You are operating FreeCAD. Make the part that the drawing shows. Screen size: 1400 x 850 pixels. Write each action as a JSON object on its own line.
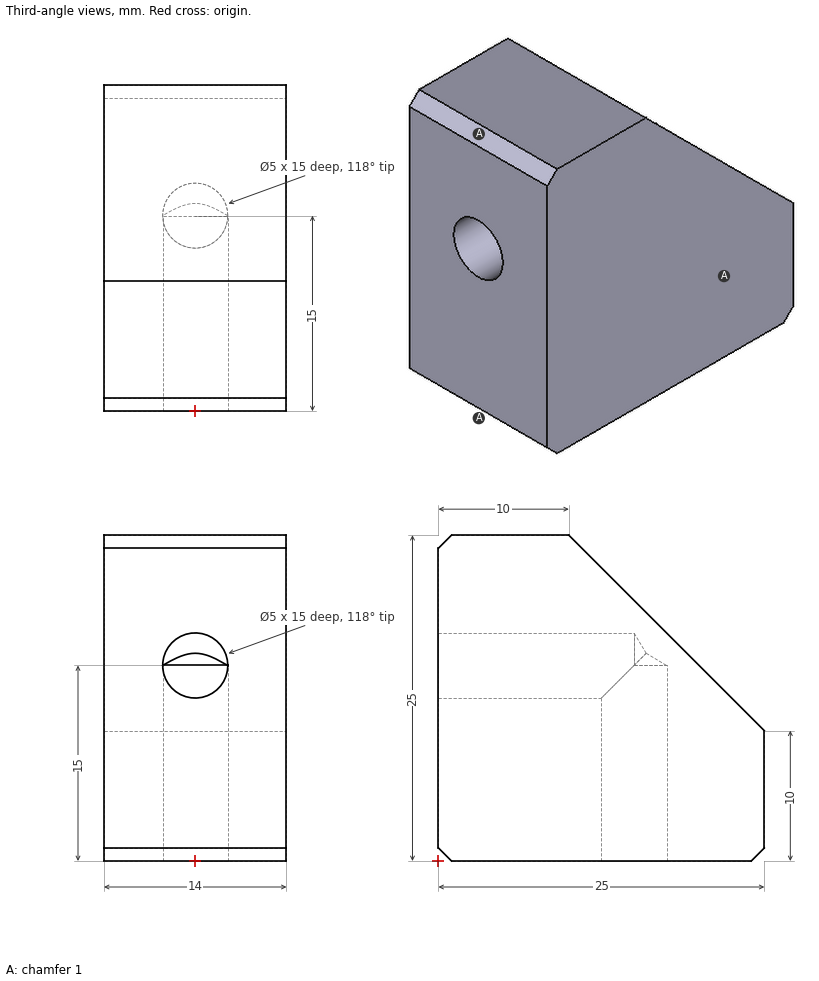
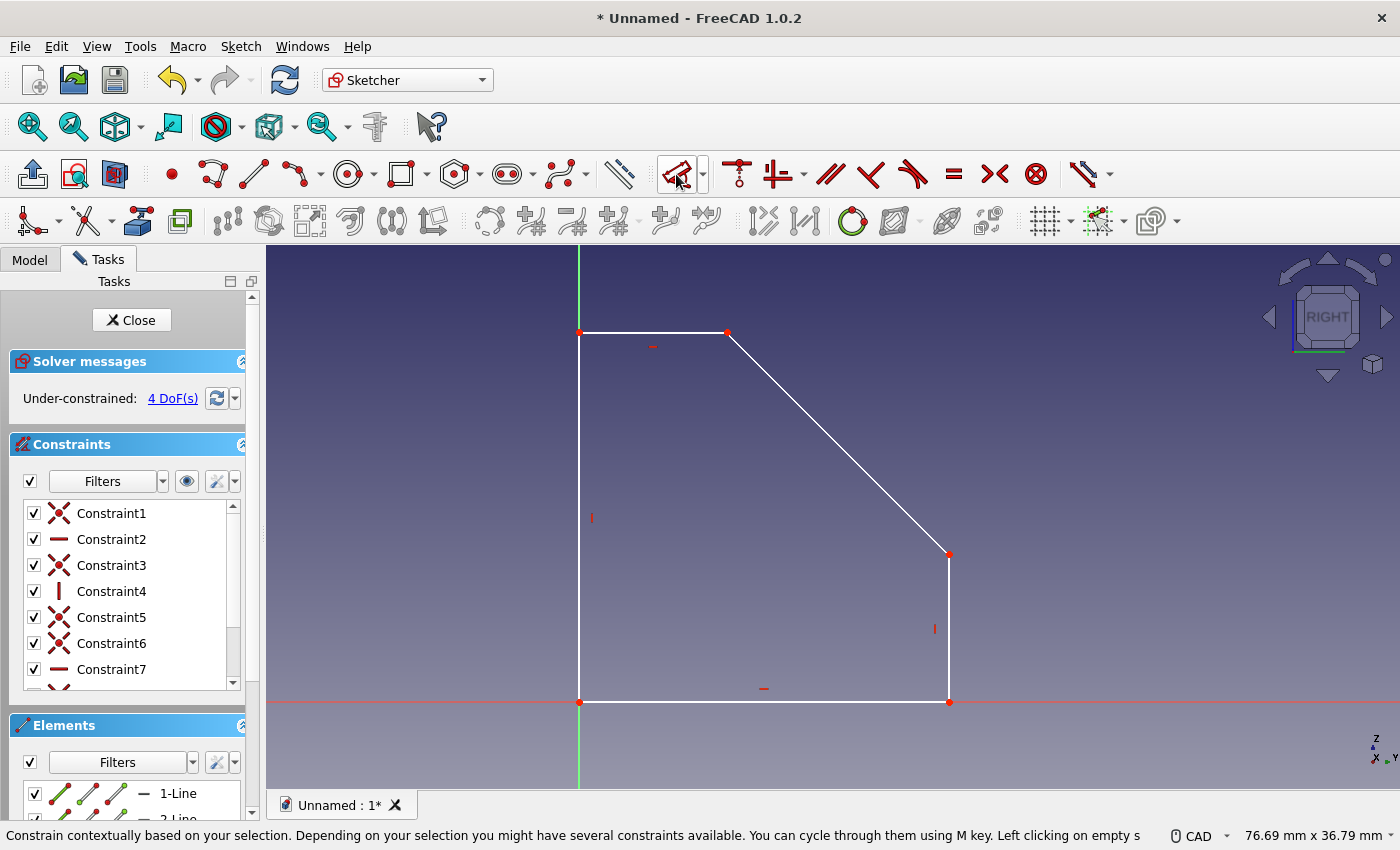
{"action": "left_click", "coordinate": [690, 702]}
{"action": "left_click", "coordinate": [764, 736]}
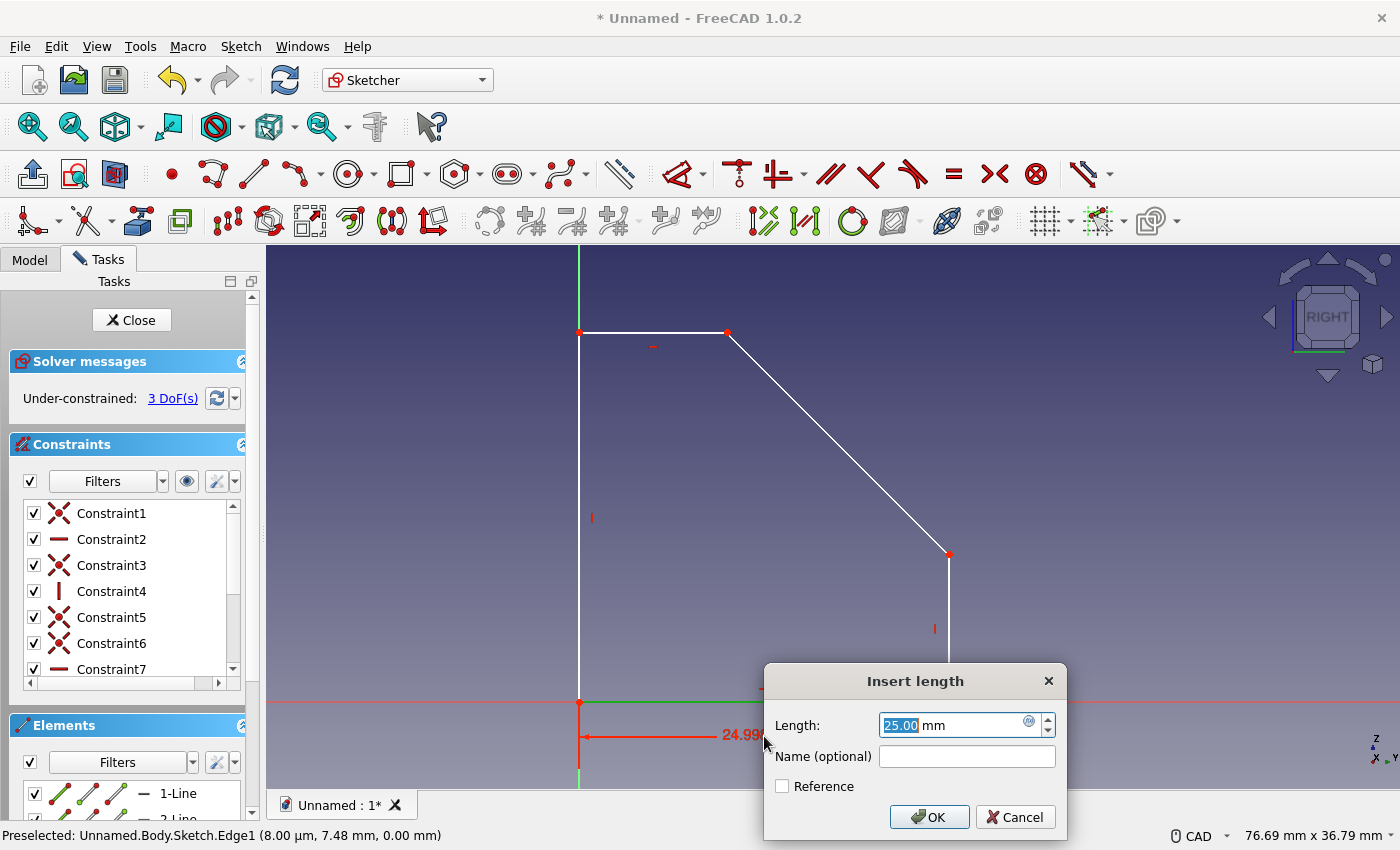
{"action": "type", "text": "25"}
{"action": "key", "text": "Return"}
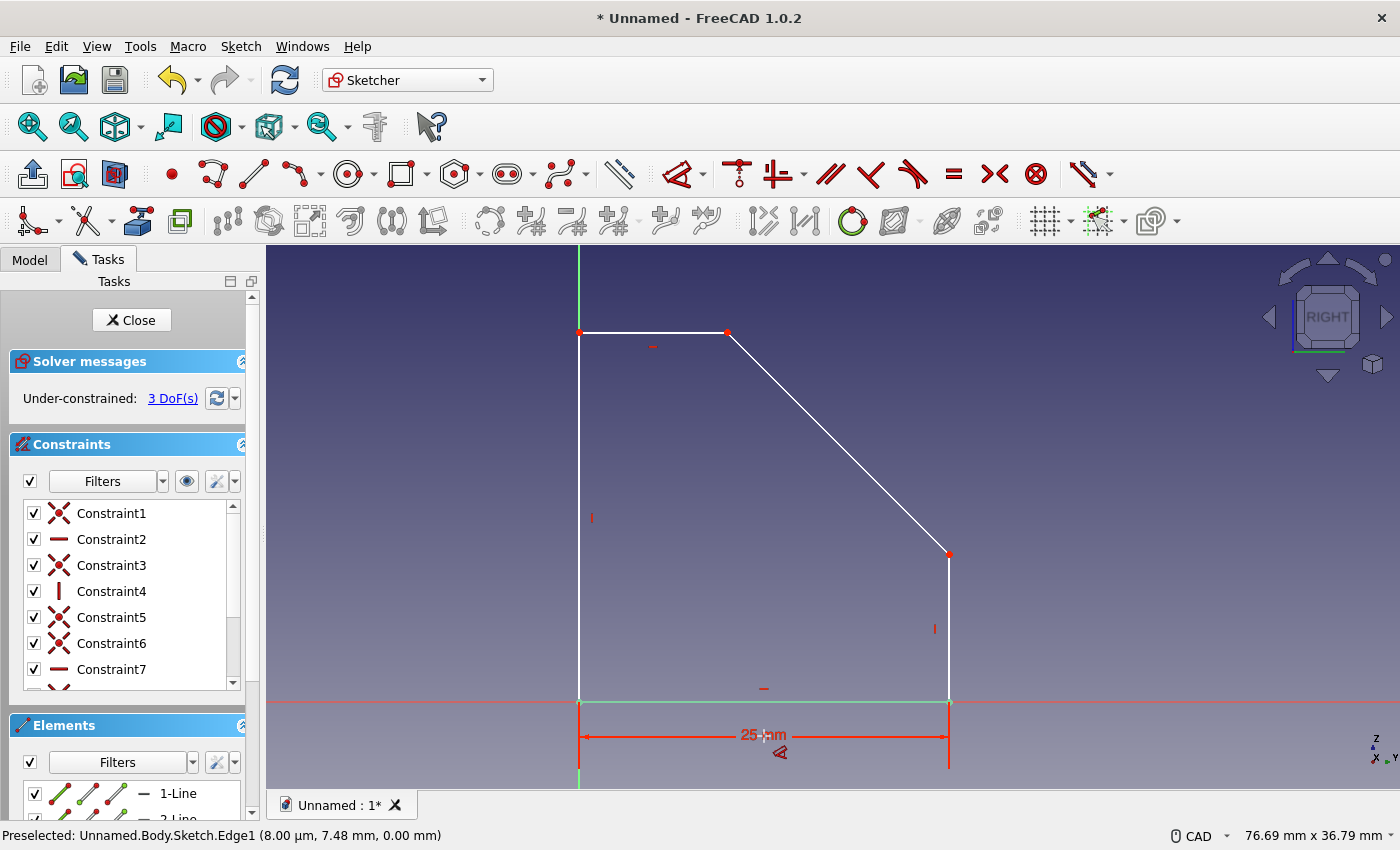
{"action": "left_click", "coordinate": [949, 658]}
{"action": "left_click", "coordinate": [983, 629]}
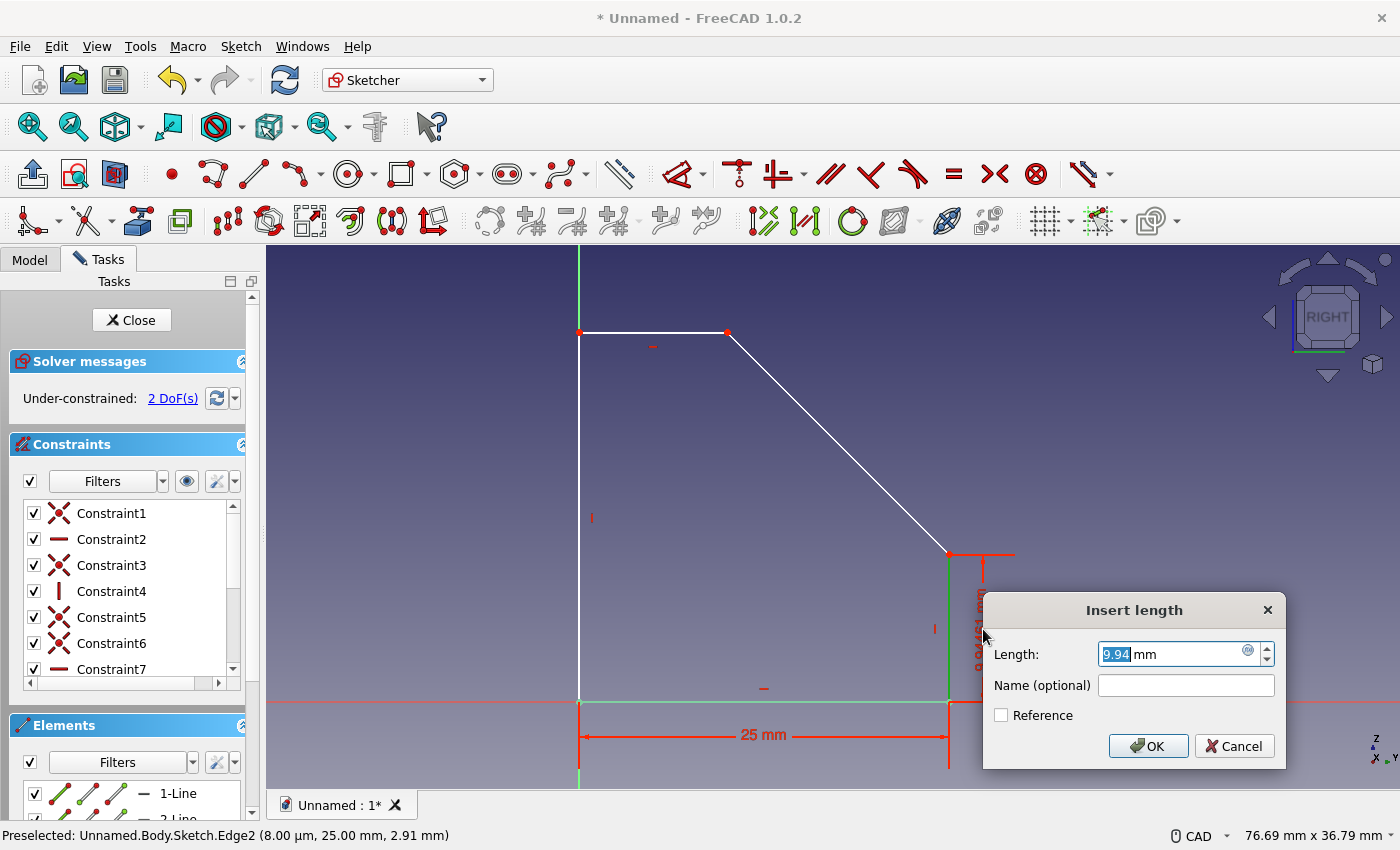
{"action": "type", "text": "10"}
{"action": "key", "text": "Return"}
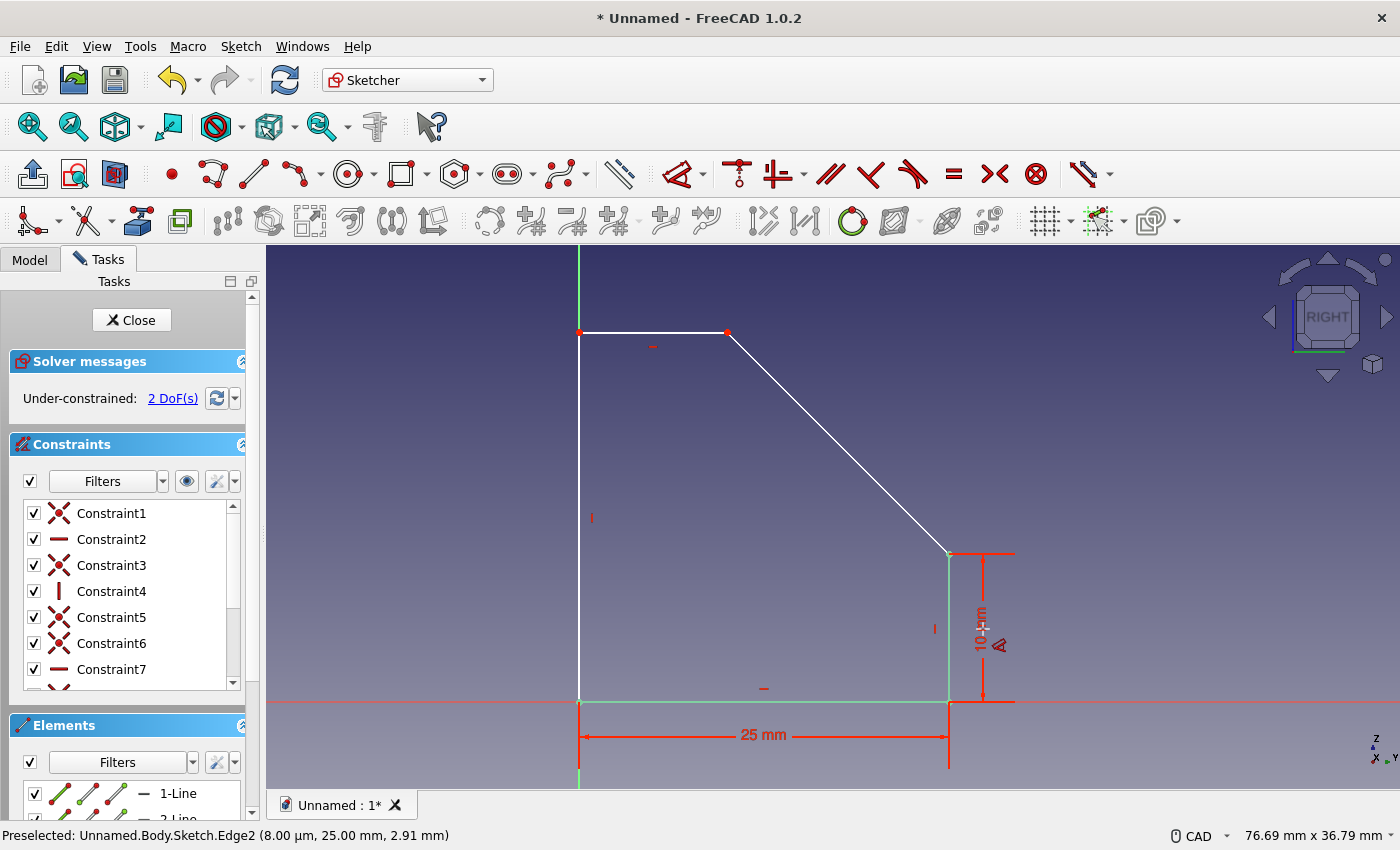
{"action": "left_click", "coordinate": [683, 333]}
{"action": "left_click", "coordinate": [653, 299]}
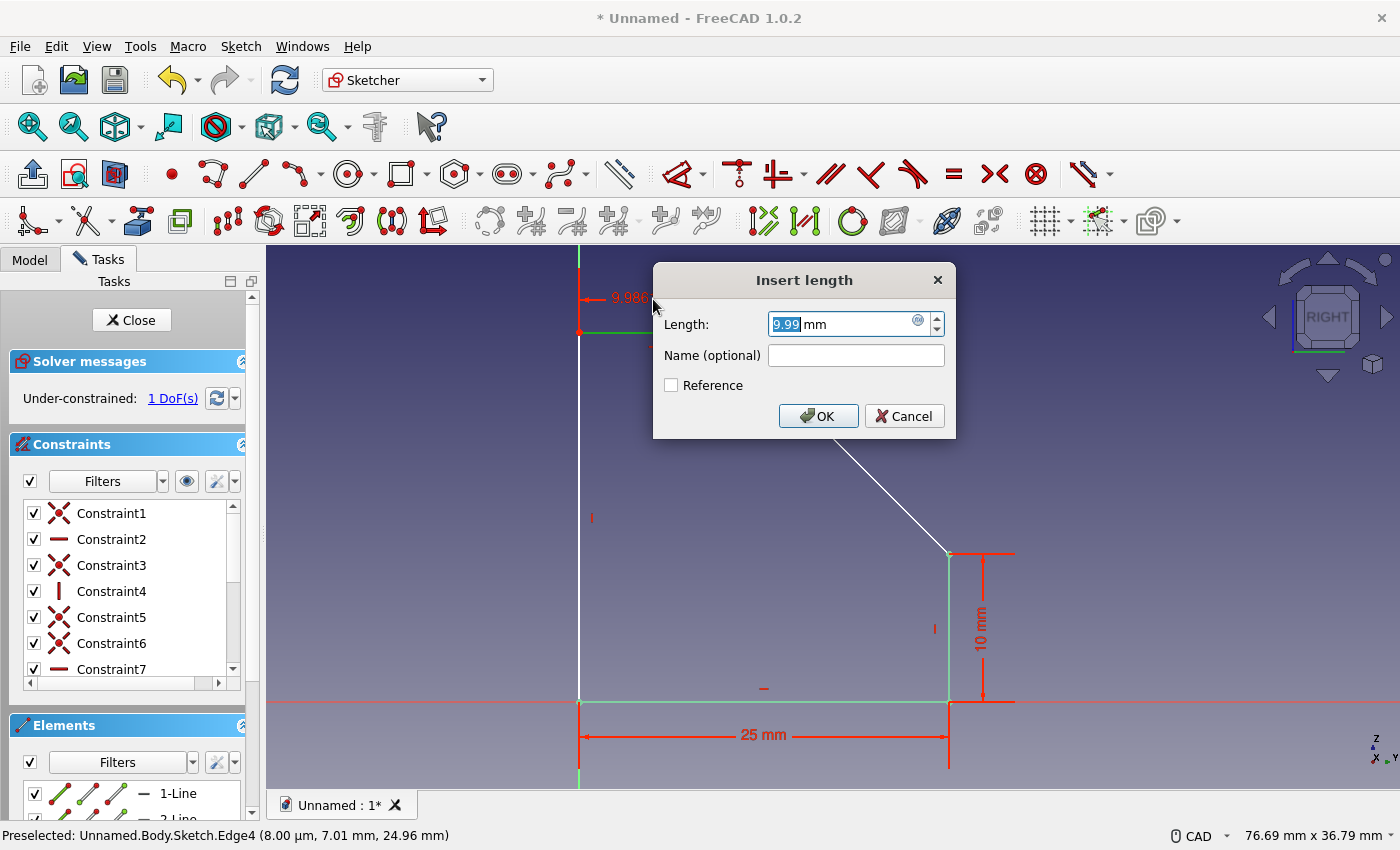
{"action": "type", "text": "10"}
{"action": "key", "text": "Return"}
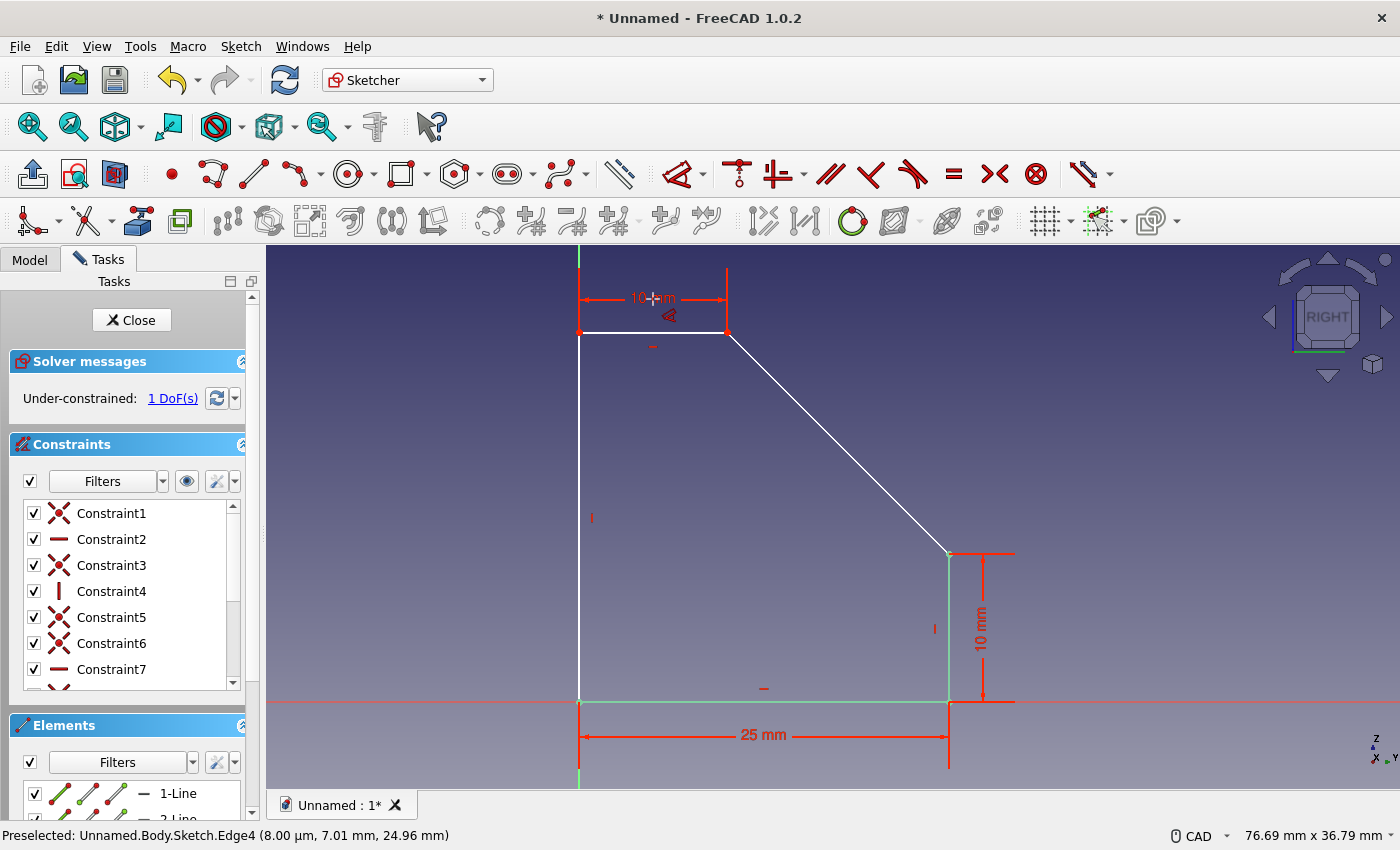
{"action": "left_click", "coordinate": [579, 444]}
{"action": "left_click", "coordinate": [545, 518]}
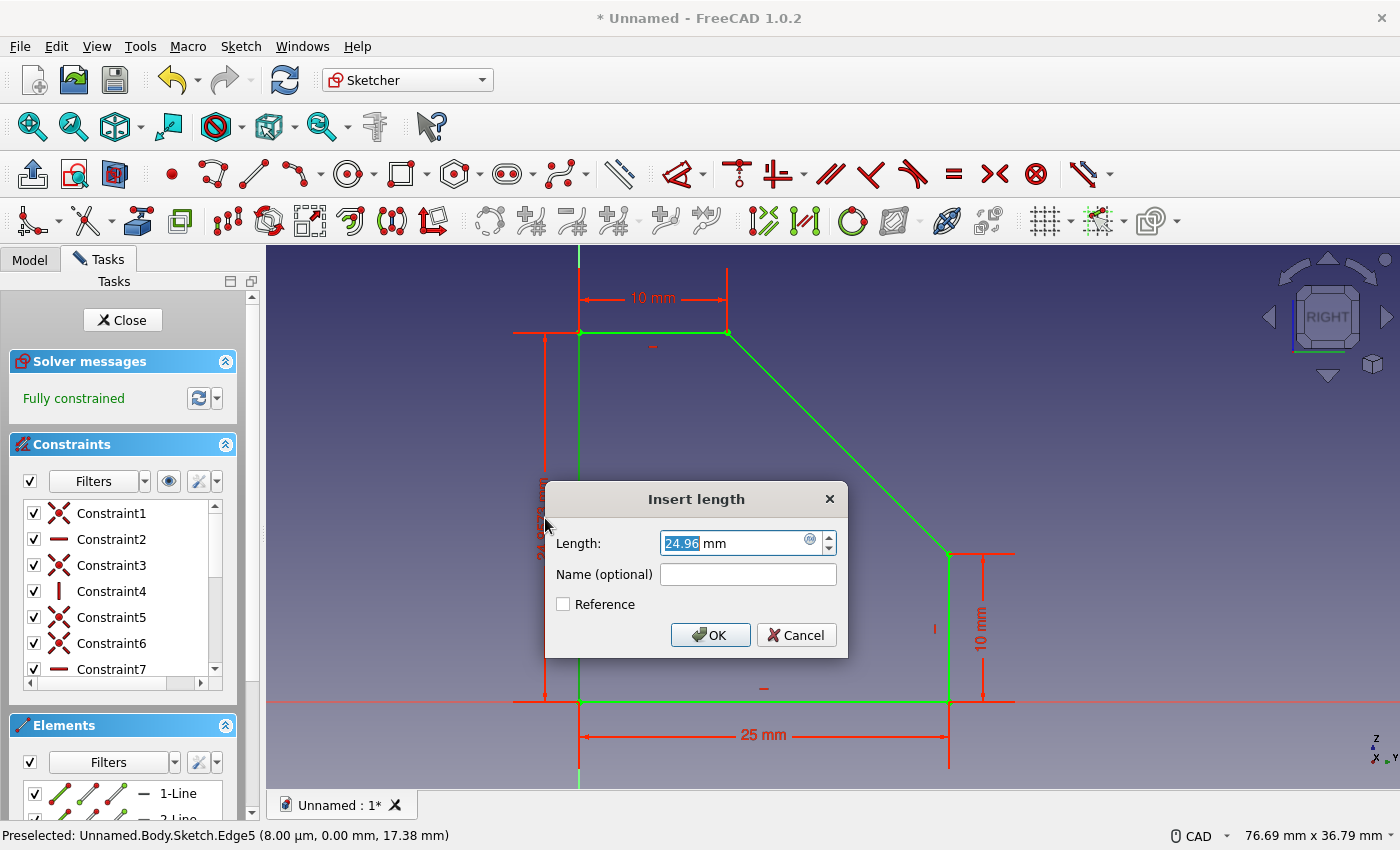
{"action": "type", "text": "25"}
{"action": "key", "text": "Return"}
{"action": "key", "text": "Escape"}